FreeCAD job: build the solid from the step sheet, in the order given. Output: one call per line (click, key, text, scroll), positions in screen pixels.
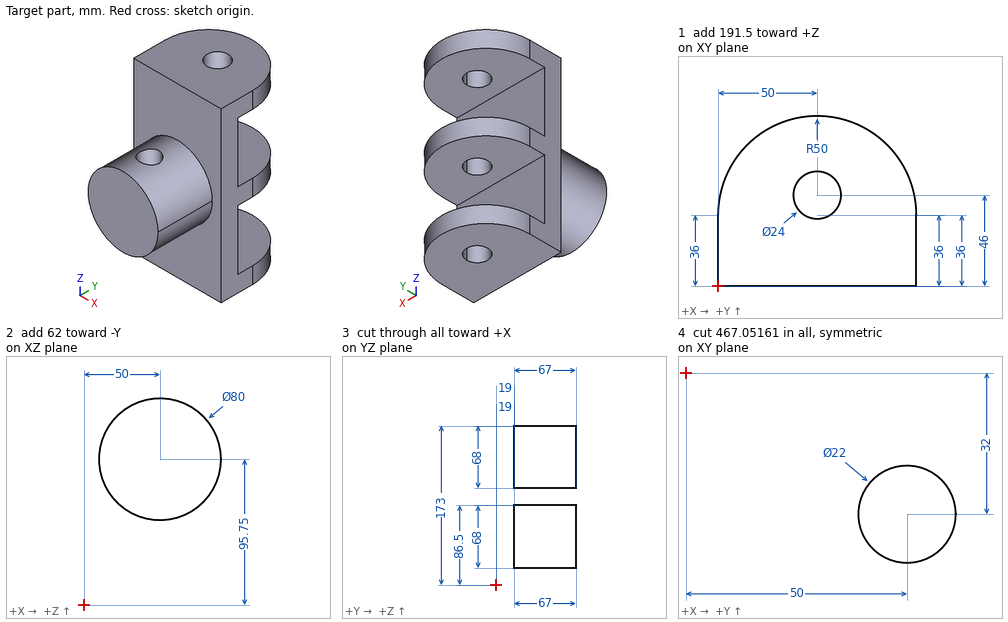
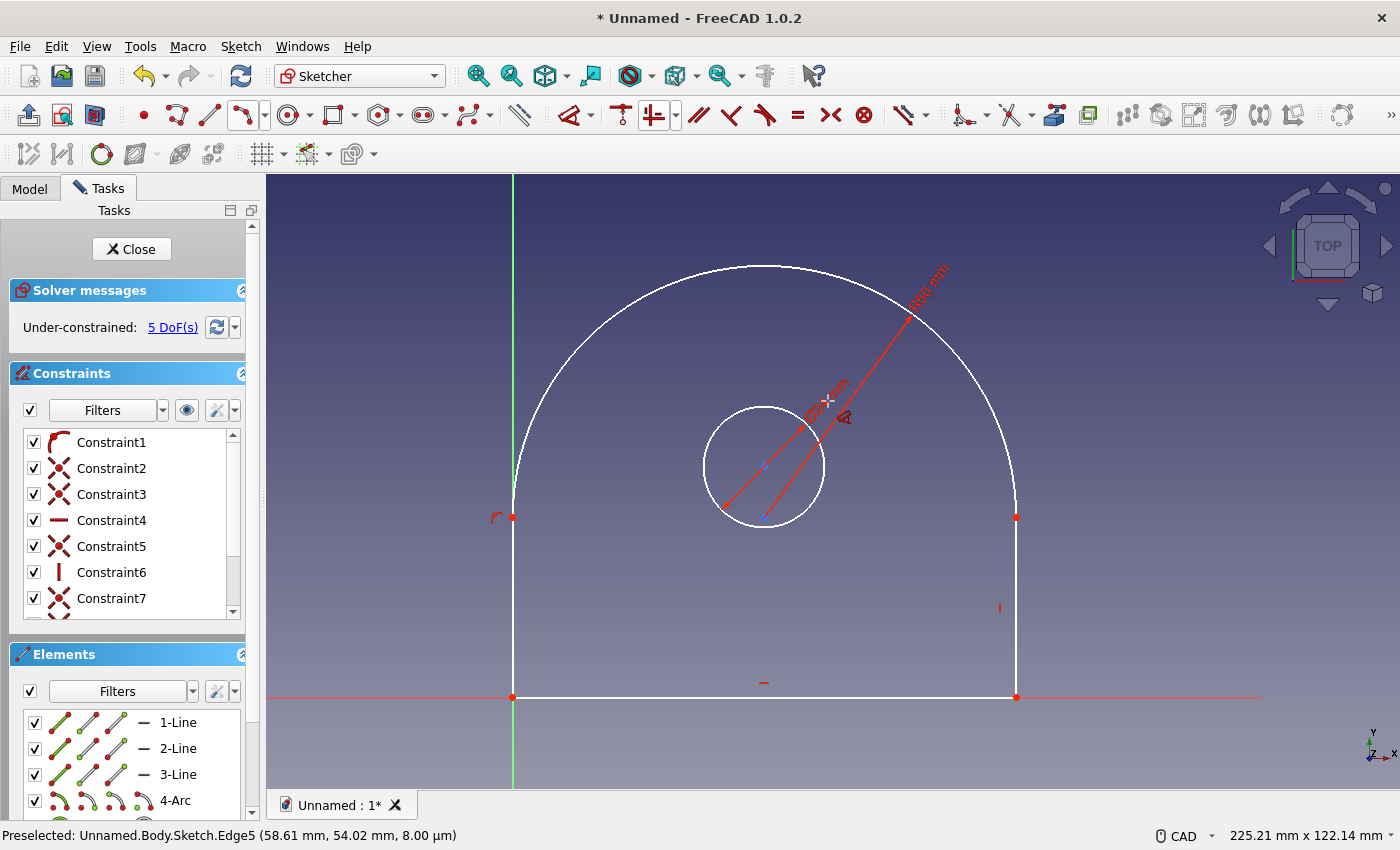
click(513, 572)
click(479, 608)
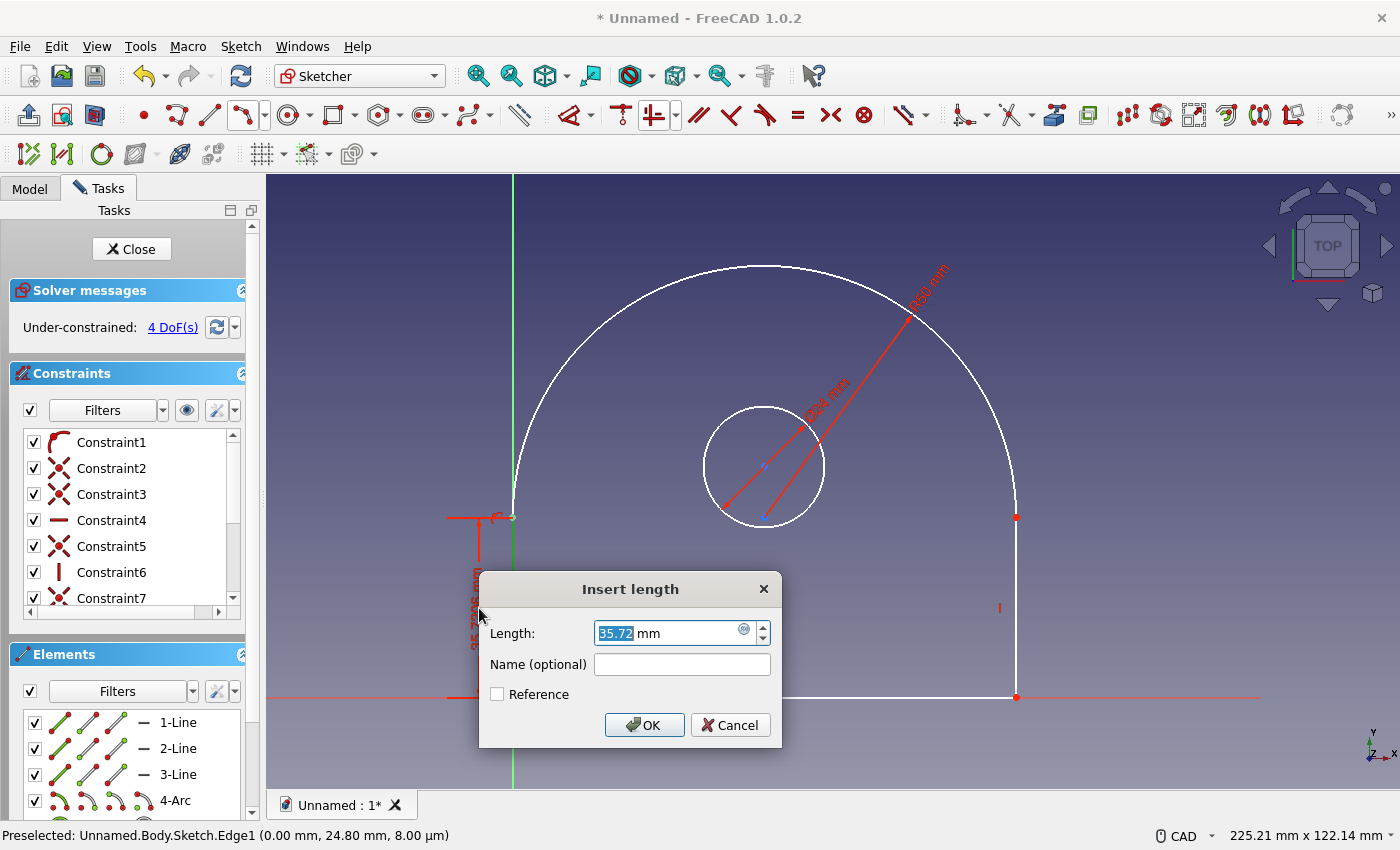
text(36)
key(Return)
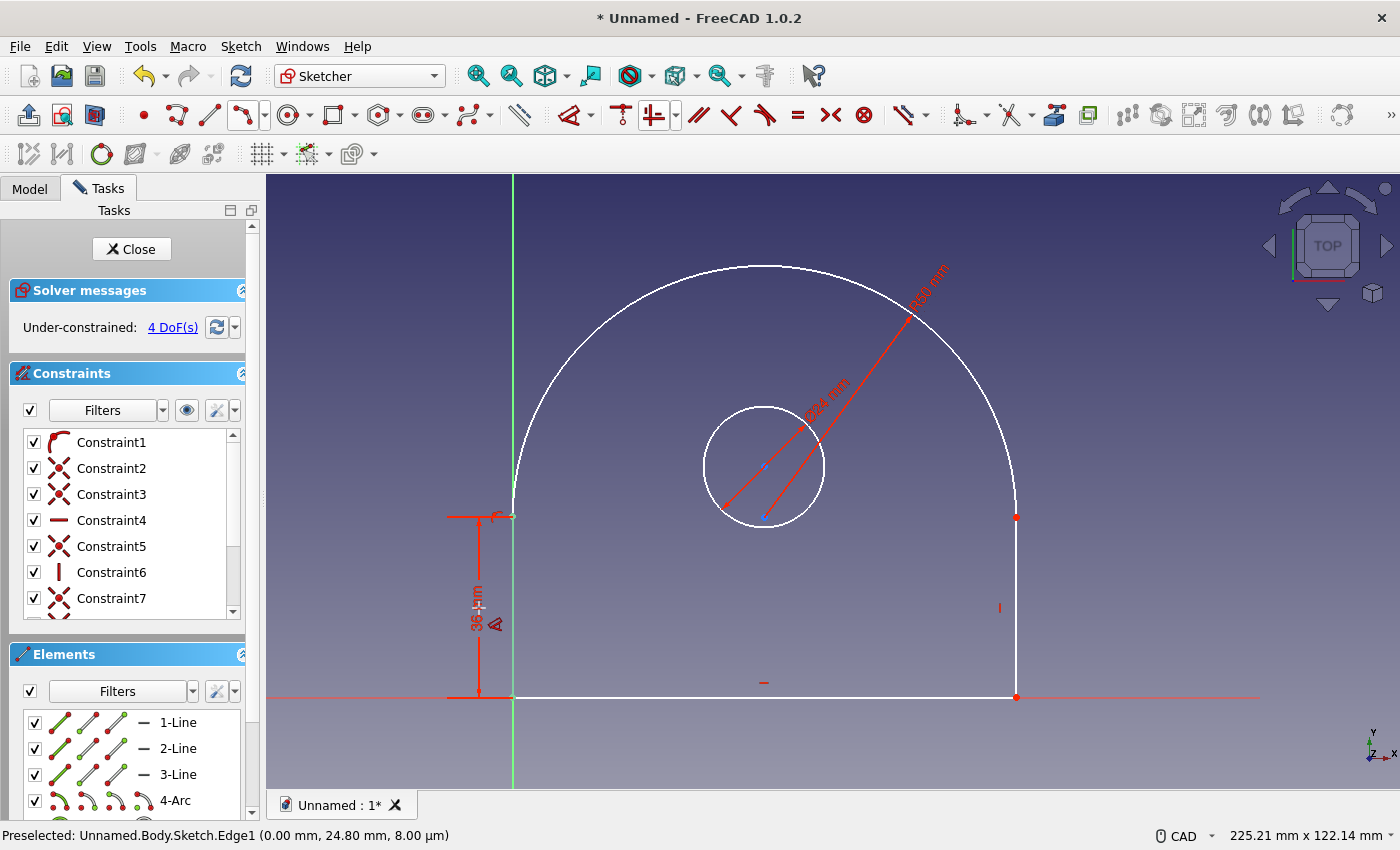
click(1016, 644)
click(1050, 608)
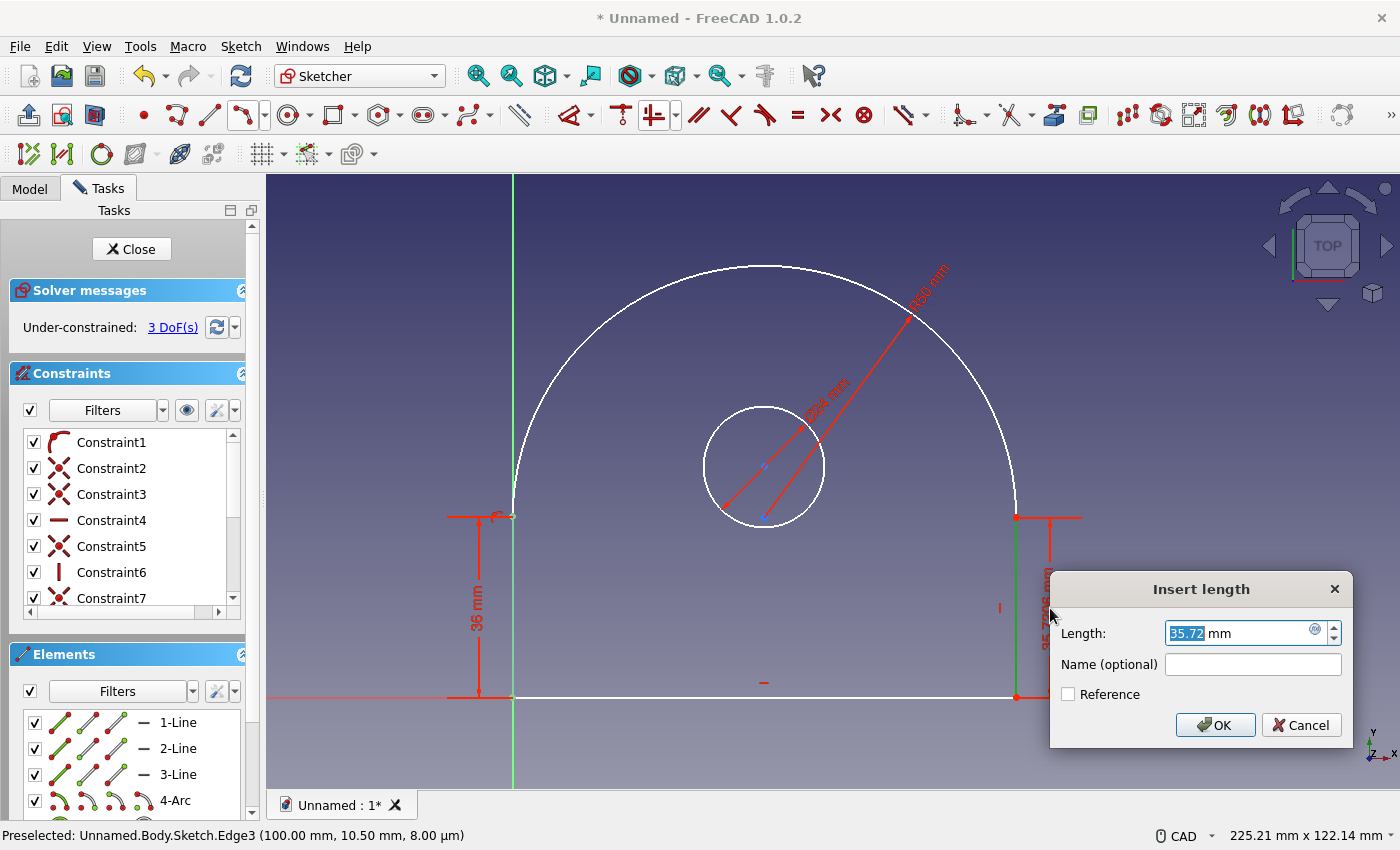
text(36)
key(Return)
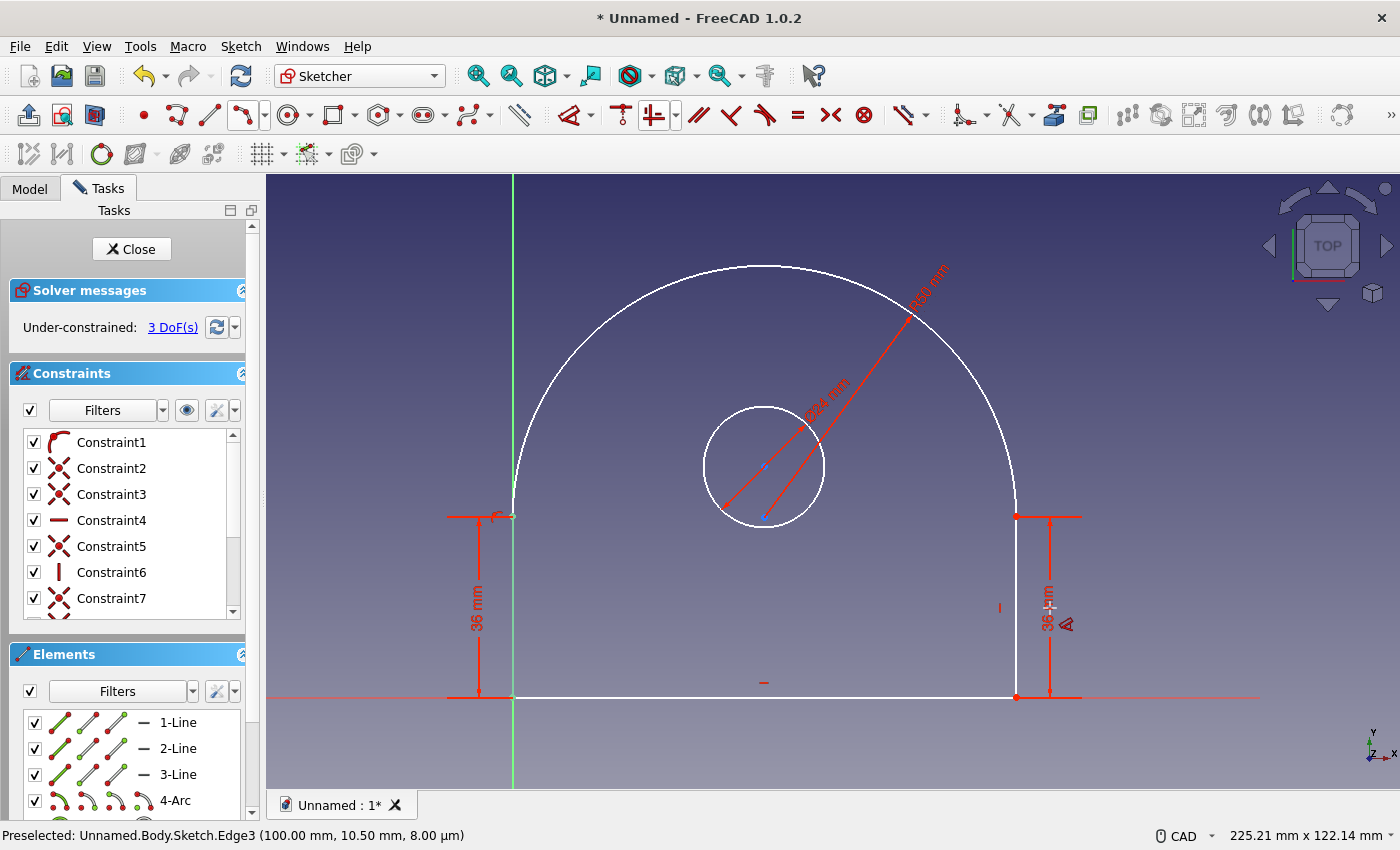
click(764, 467)
click(638, 732)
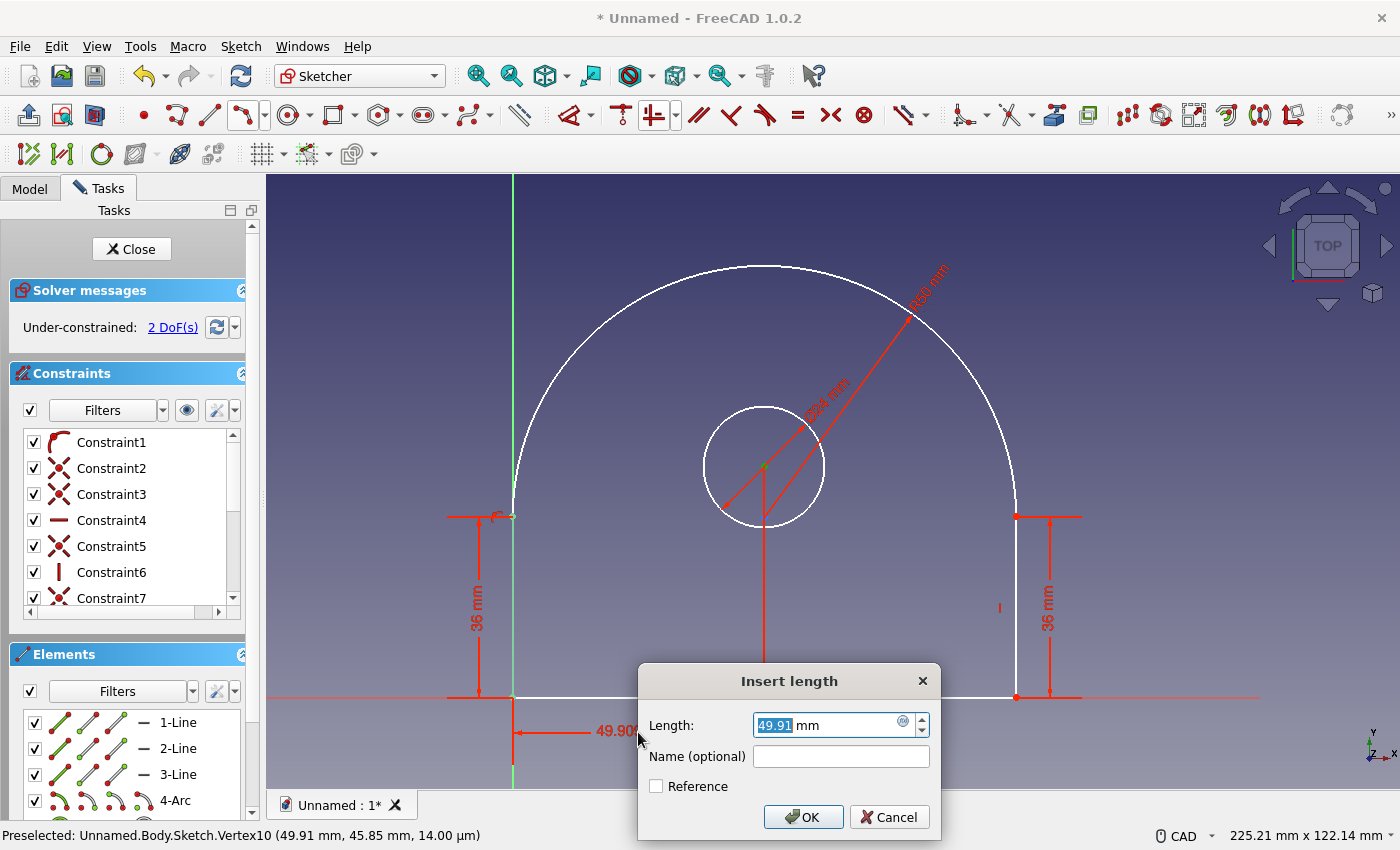
text(50)
key(Return)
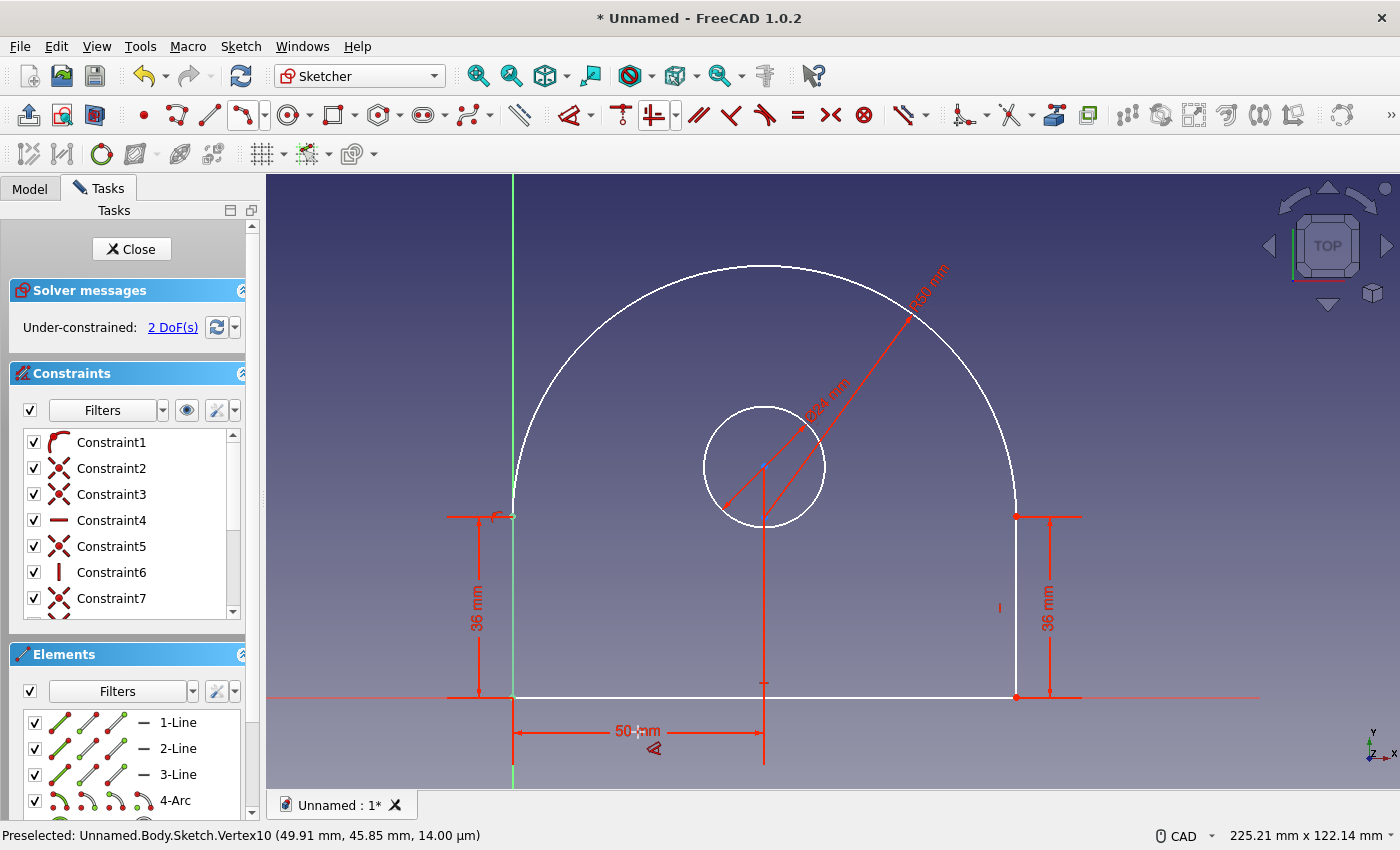
click(764, 467)
click(479, 582)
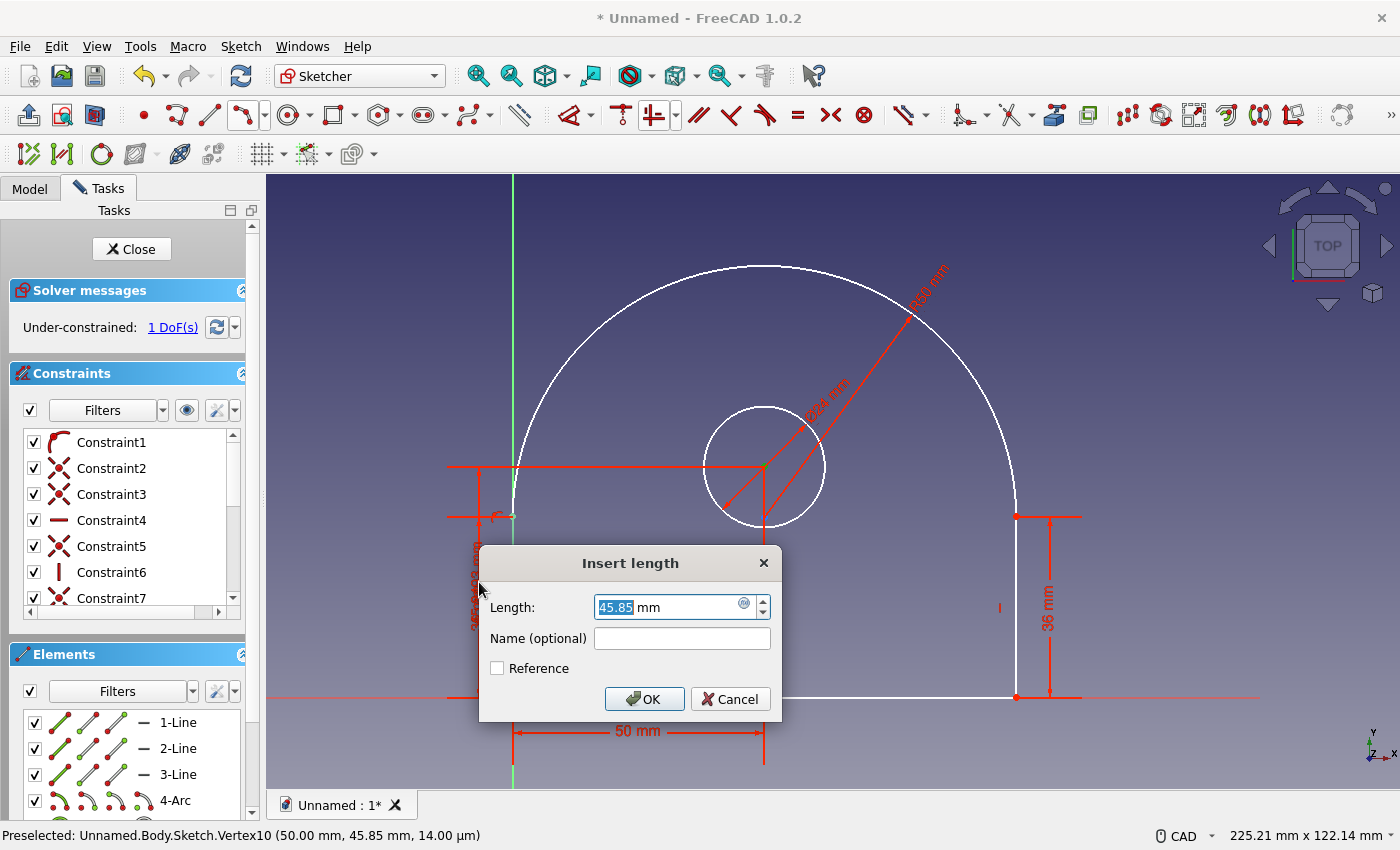
text(46)
key(Return)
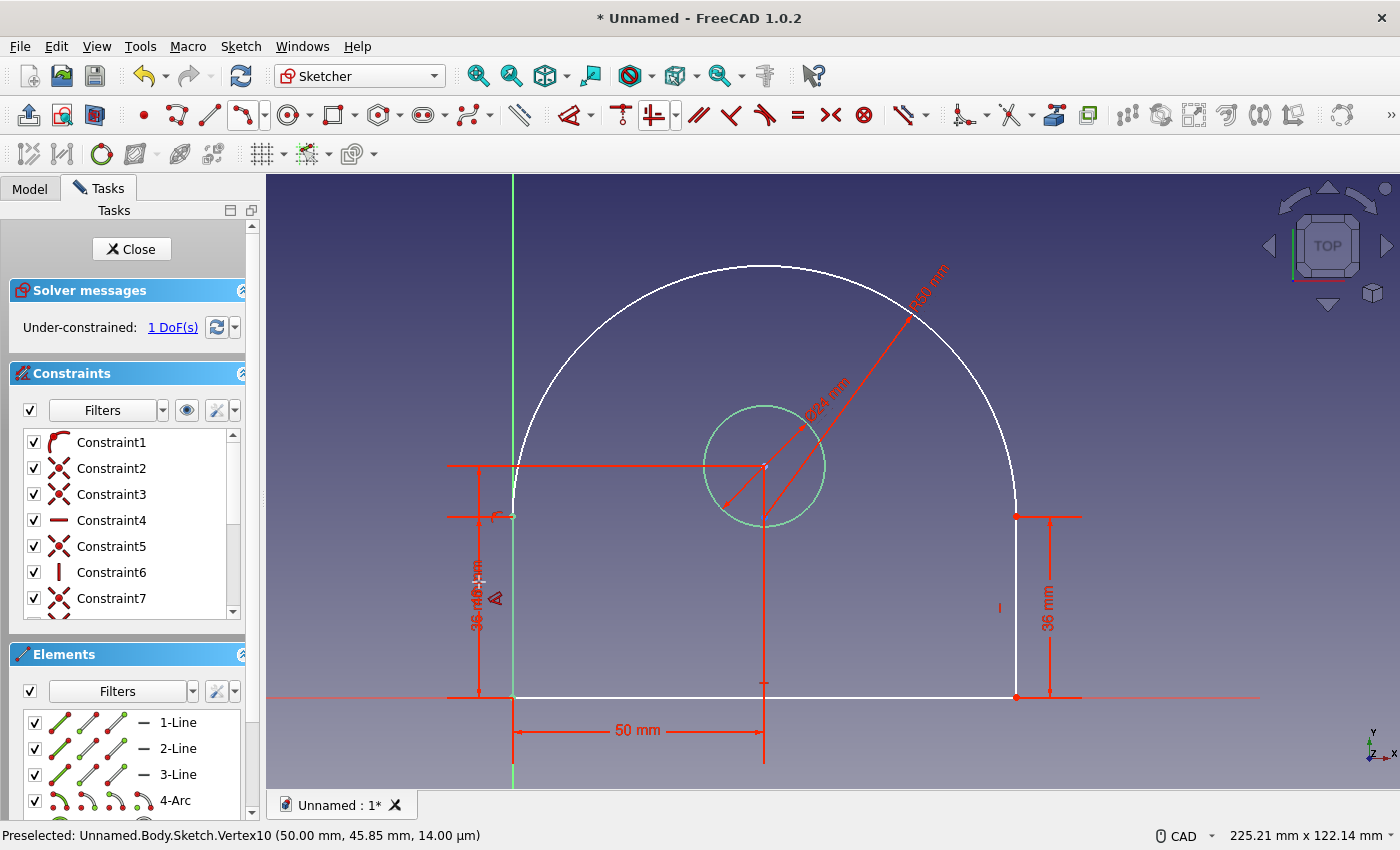
click(764, 518)
click(479, 649)